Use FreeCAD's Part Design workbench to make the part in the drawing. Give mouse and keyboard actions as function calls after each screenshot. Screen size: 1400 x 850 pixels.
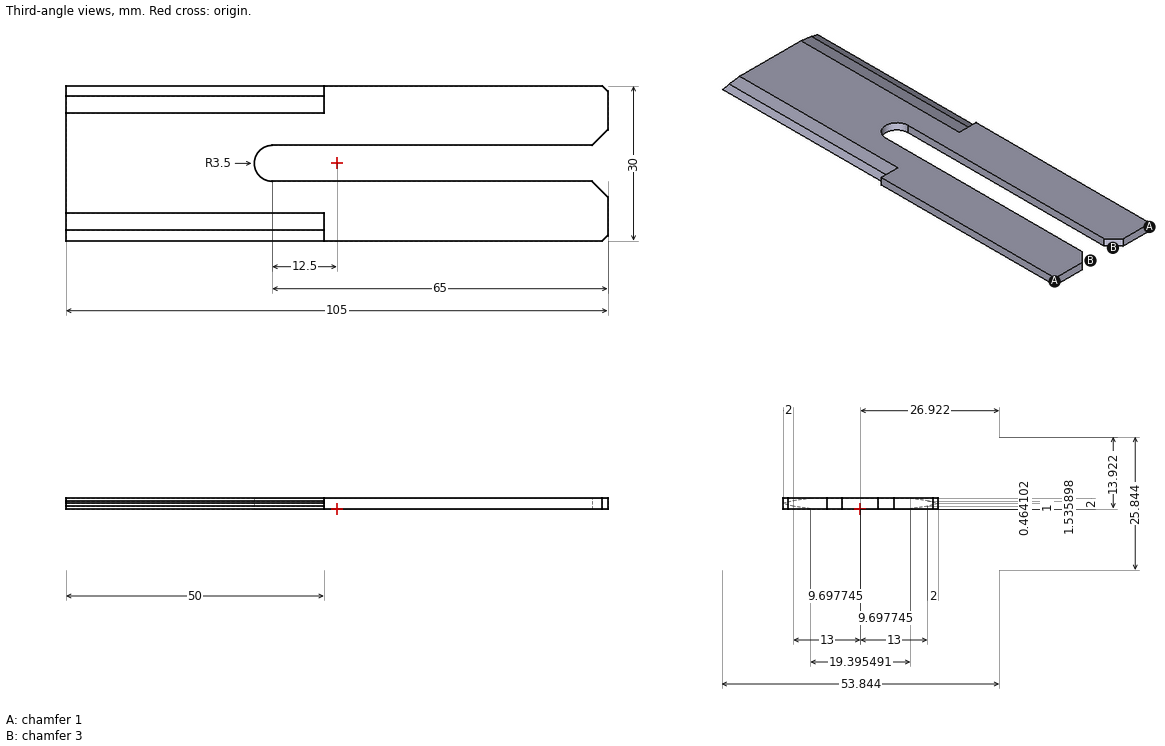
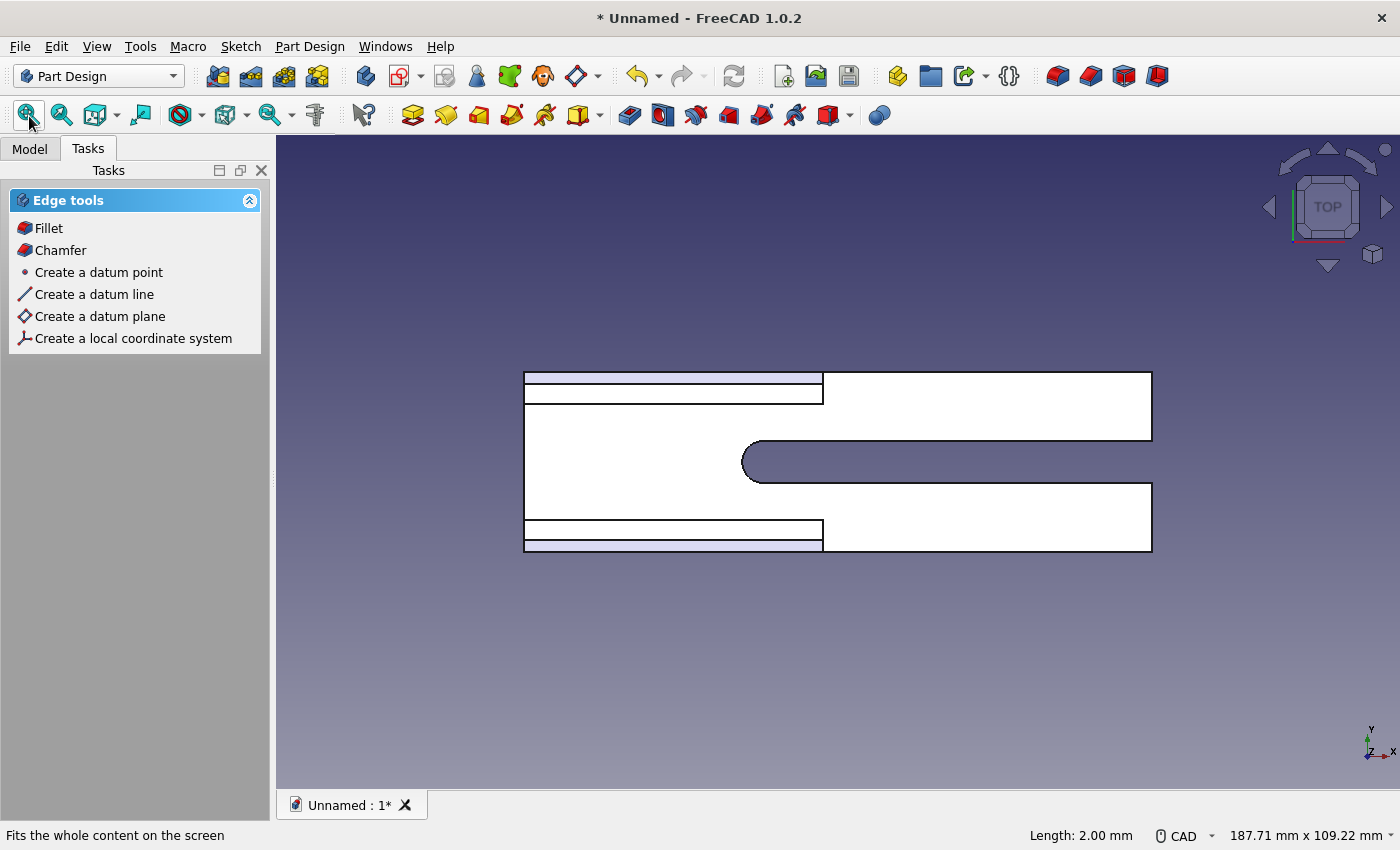
key(1)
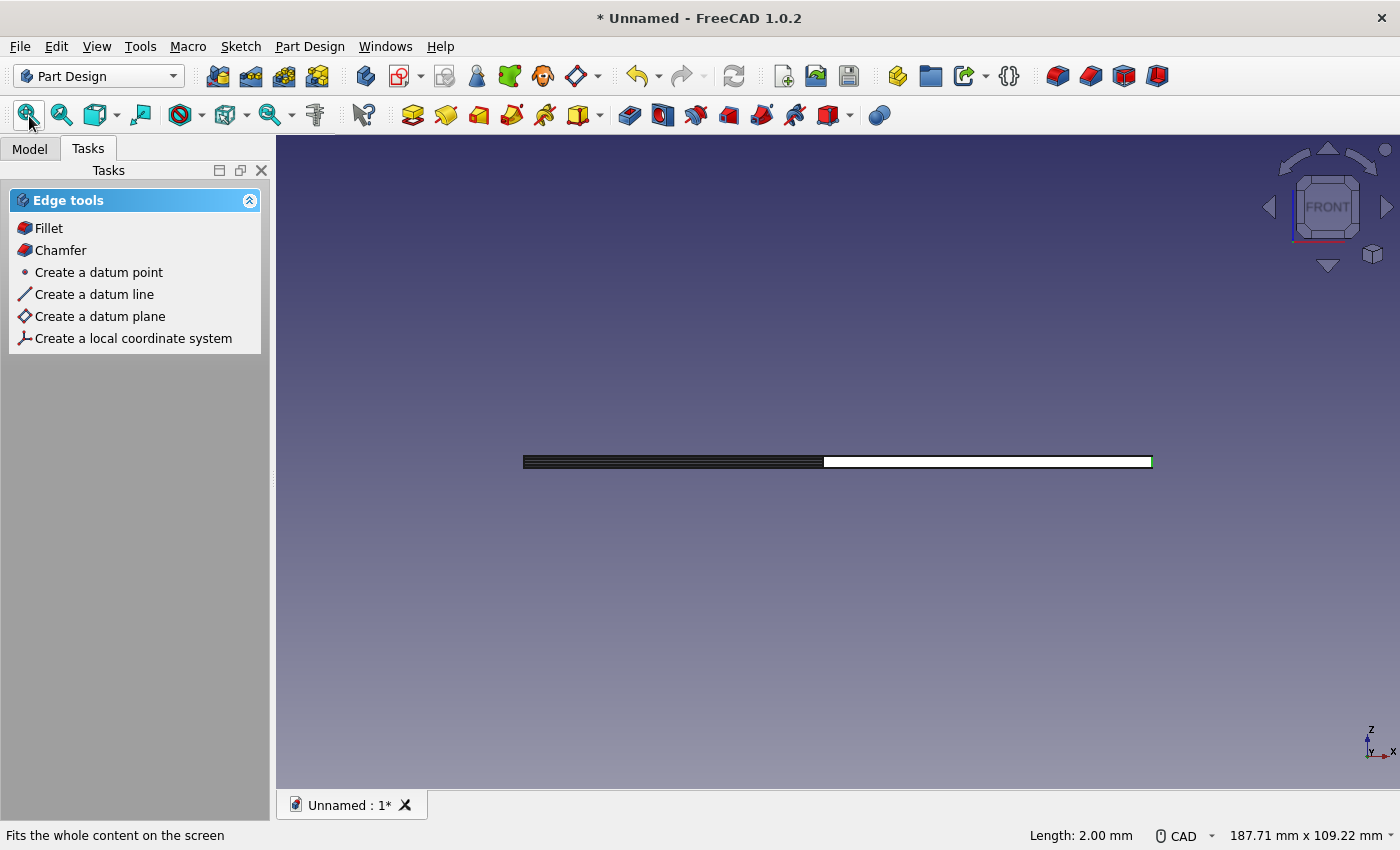
scroll(1152, 461, up, 7)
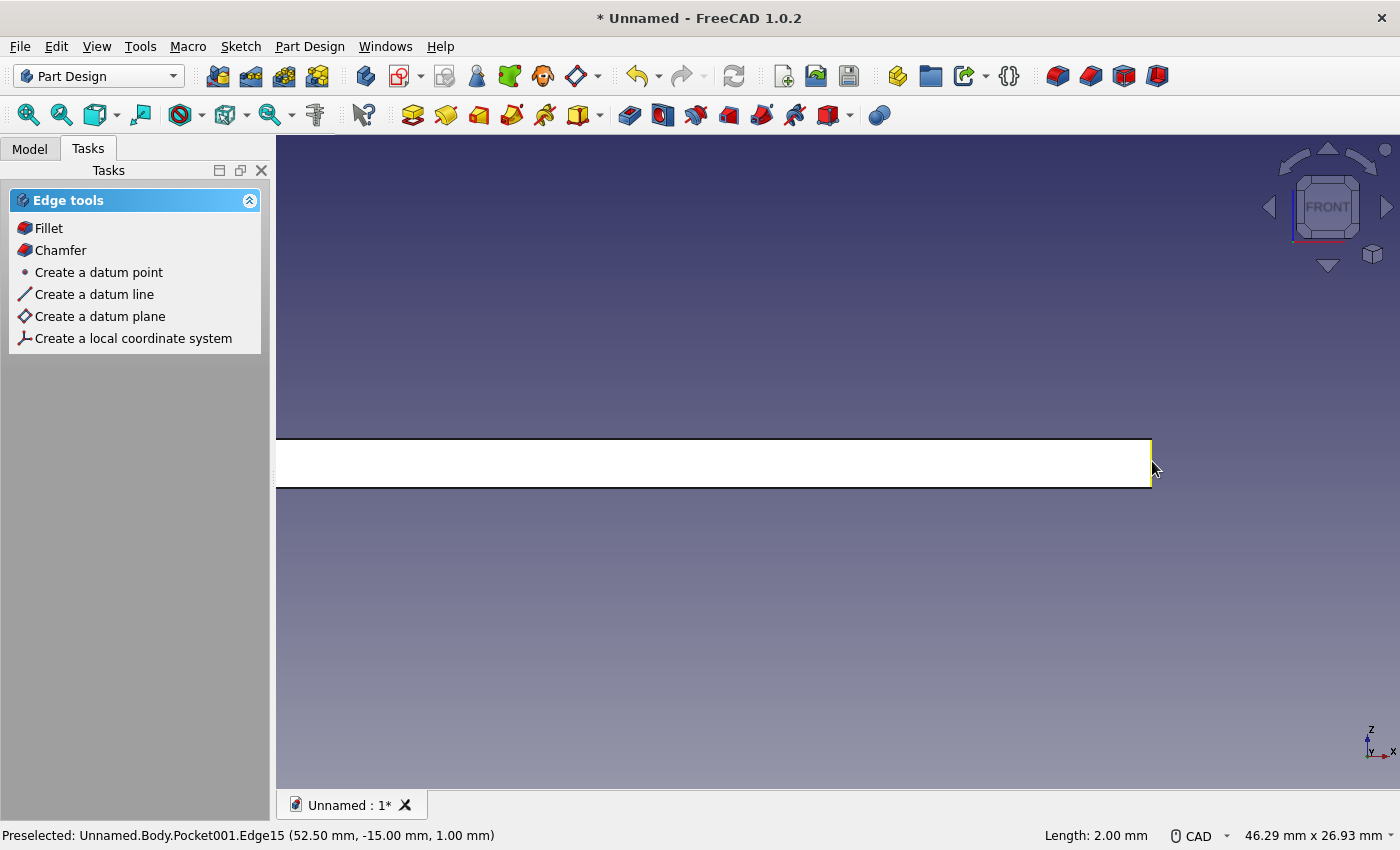
click(29, 116)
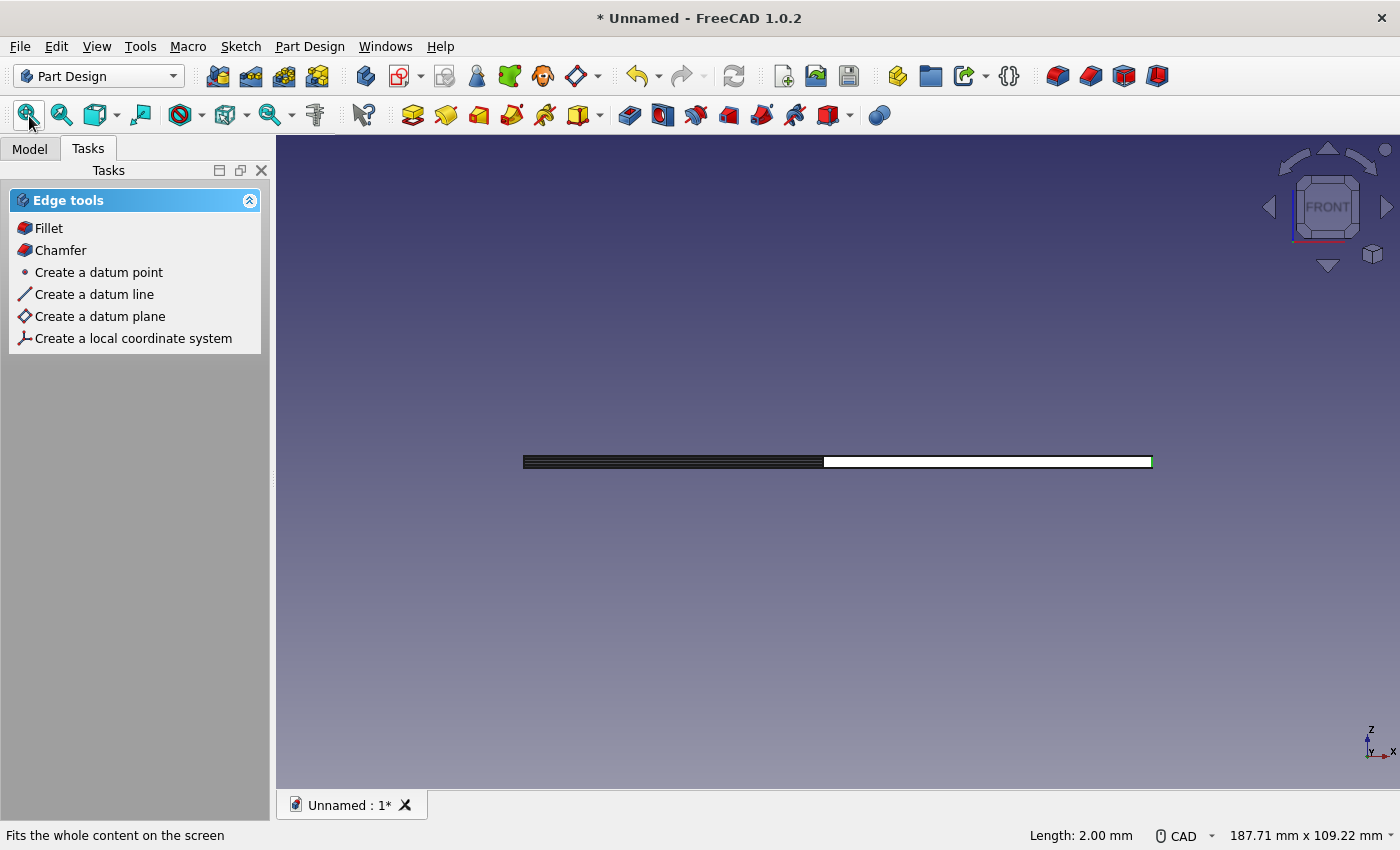
key(3)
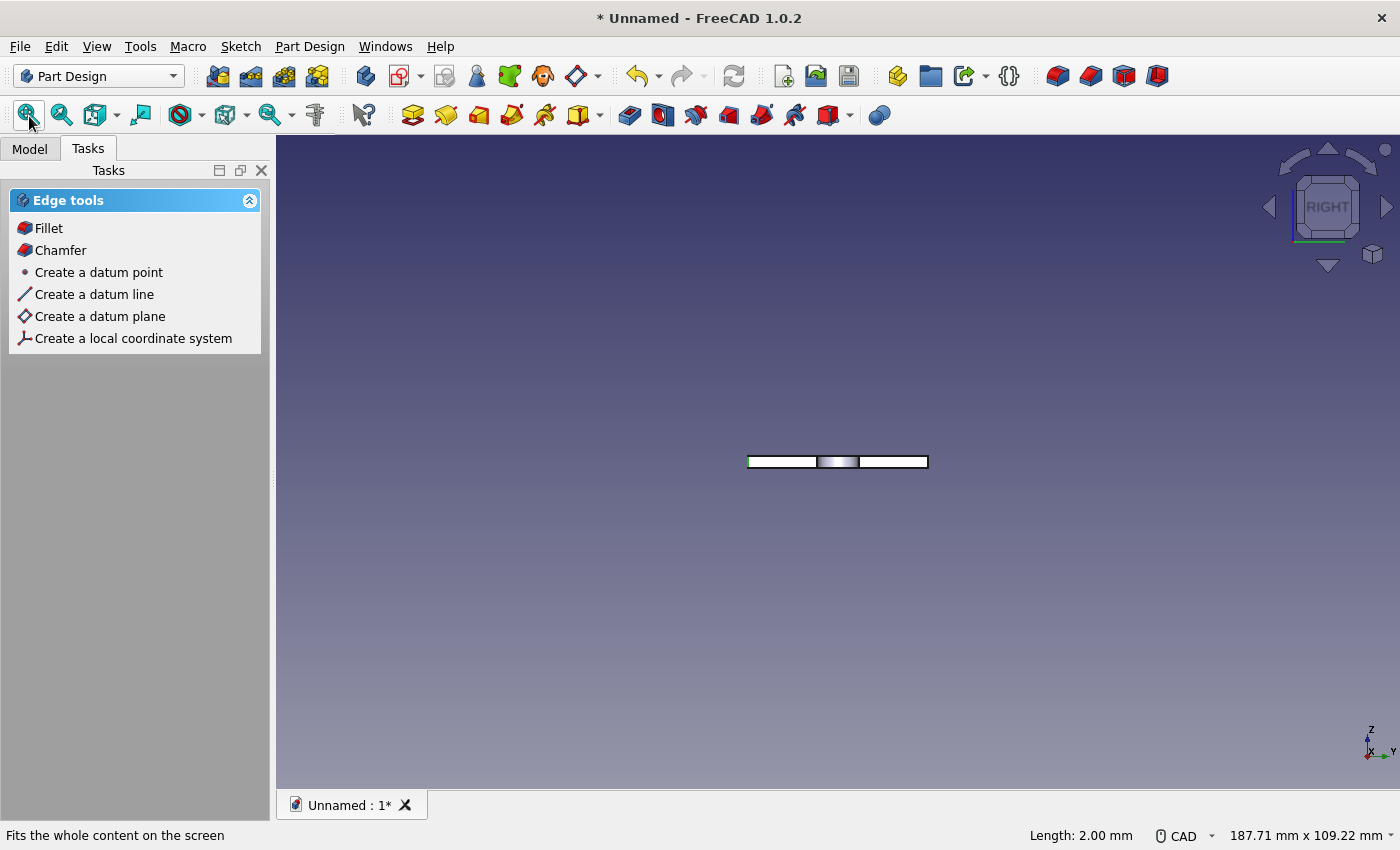
click(29, 116)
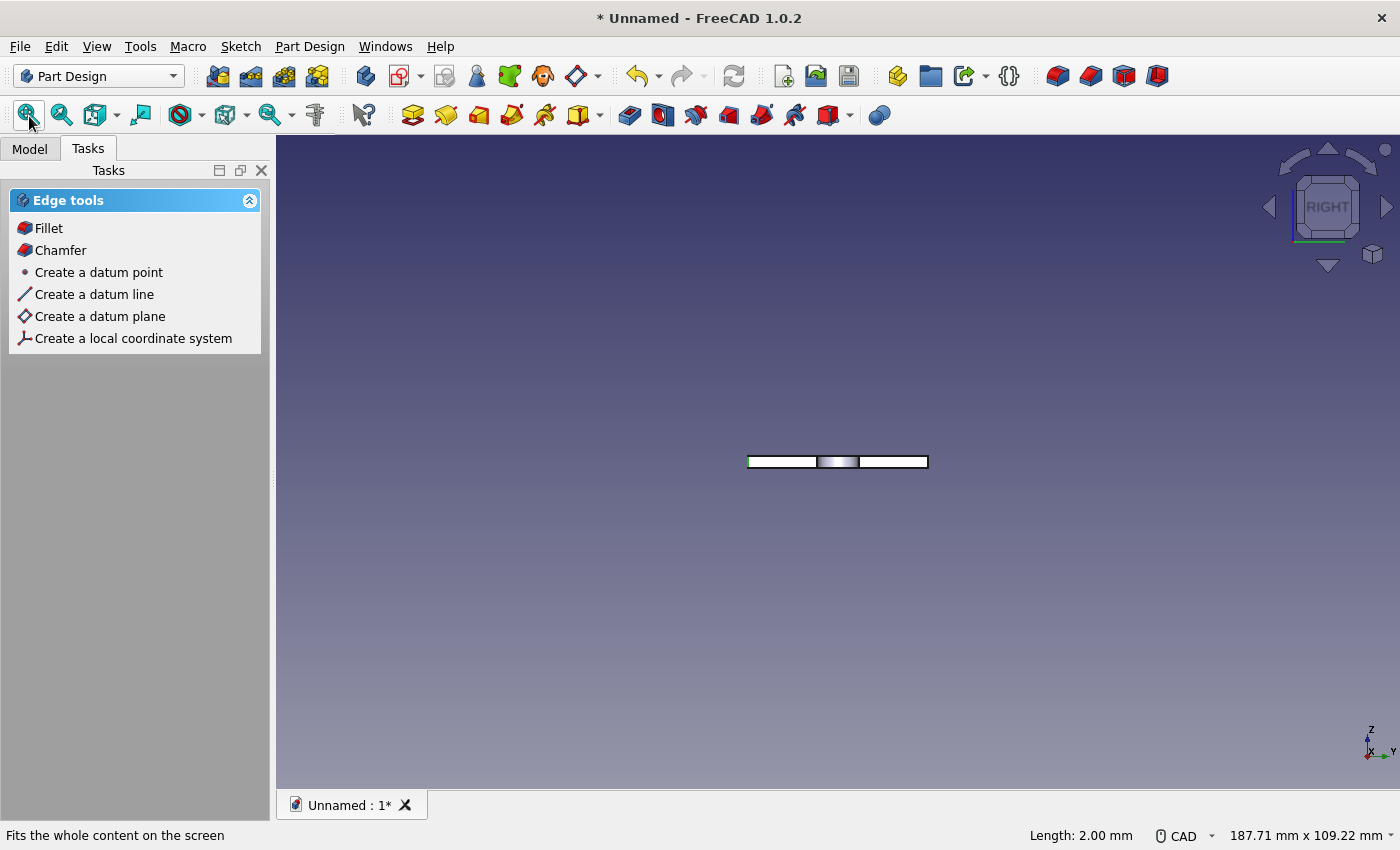
click(928, 461, ctrl)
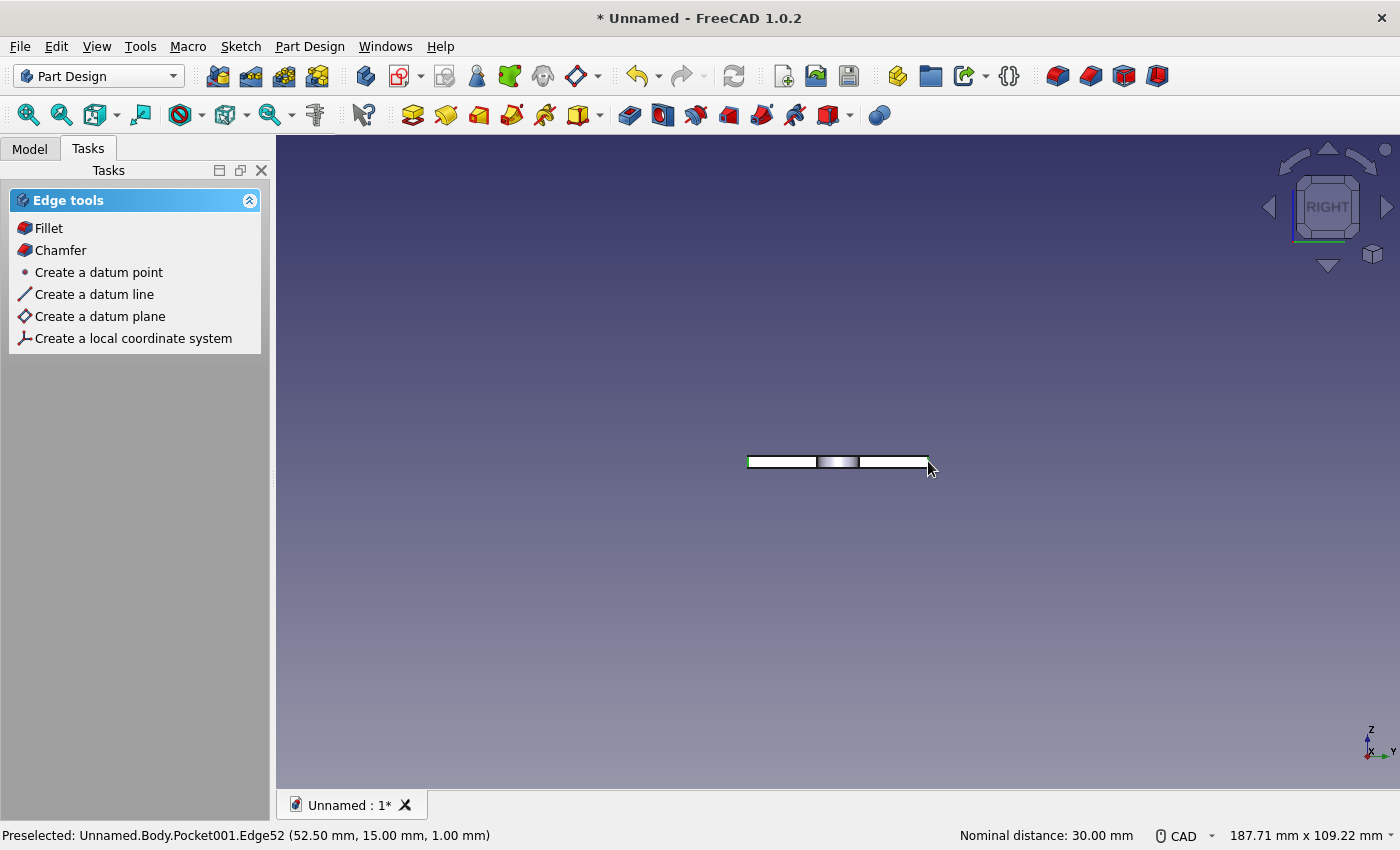
click(1091, 76)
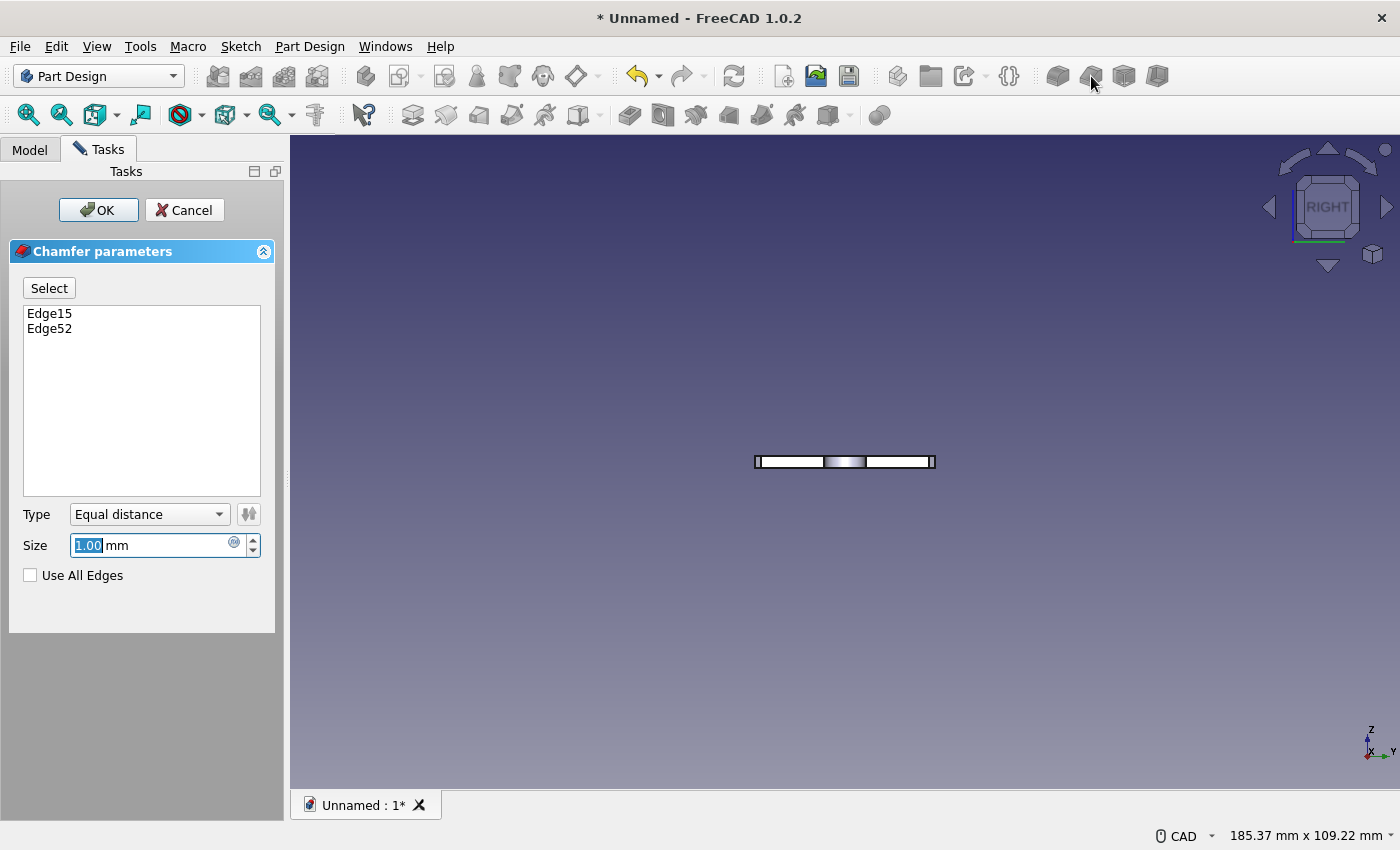
text(1)
key(Tab)